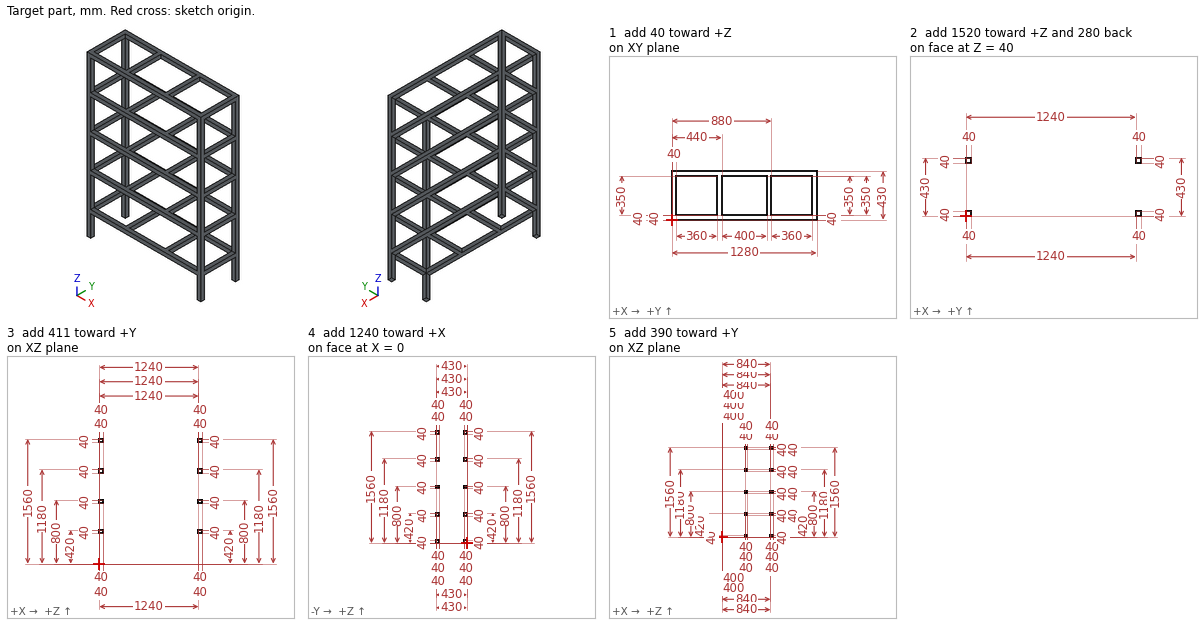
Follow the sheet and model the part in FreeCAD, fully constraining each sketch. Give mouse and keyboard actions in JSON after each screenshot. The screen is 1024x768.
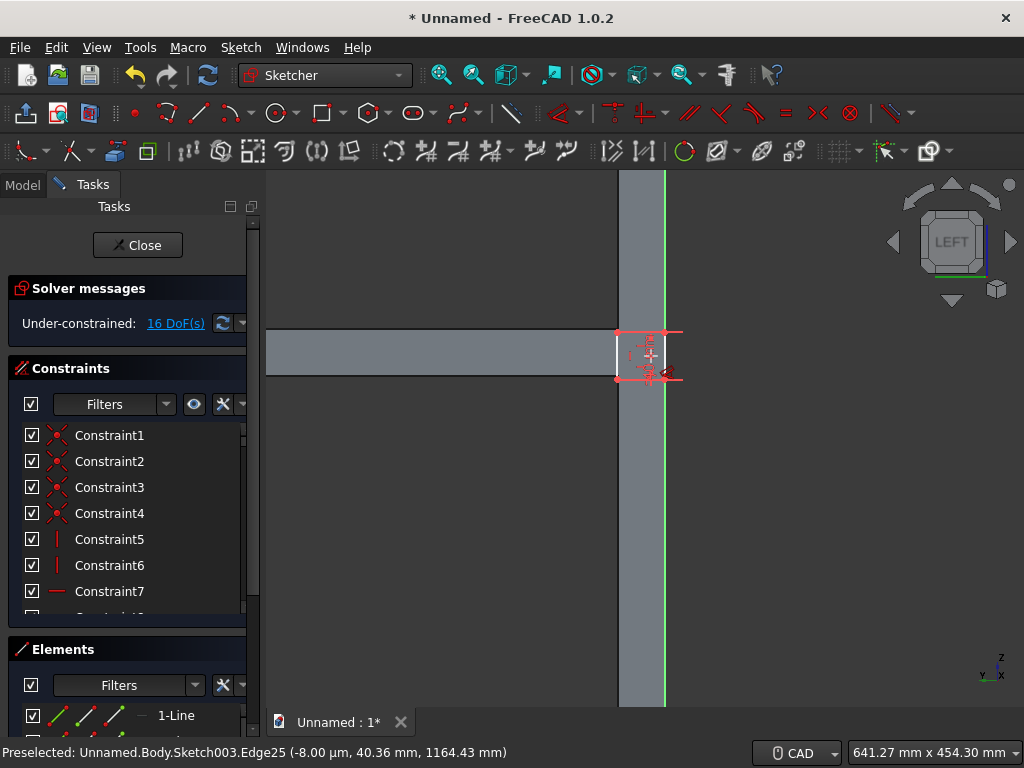
{"action": "left_click", "coordinate": [632, 380]}
{"action": "left_click", "coordinate": [641, 414]}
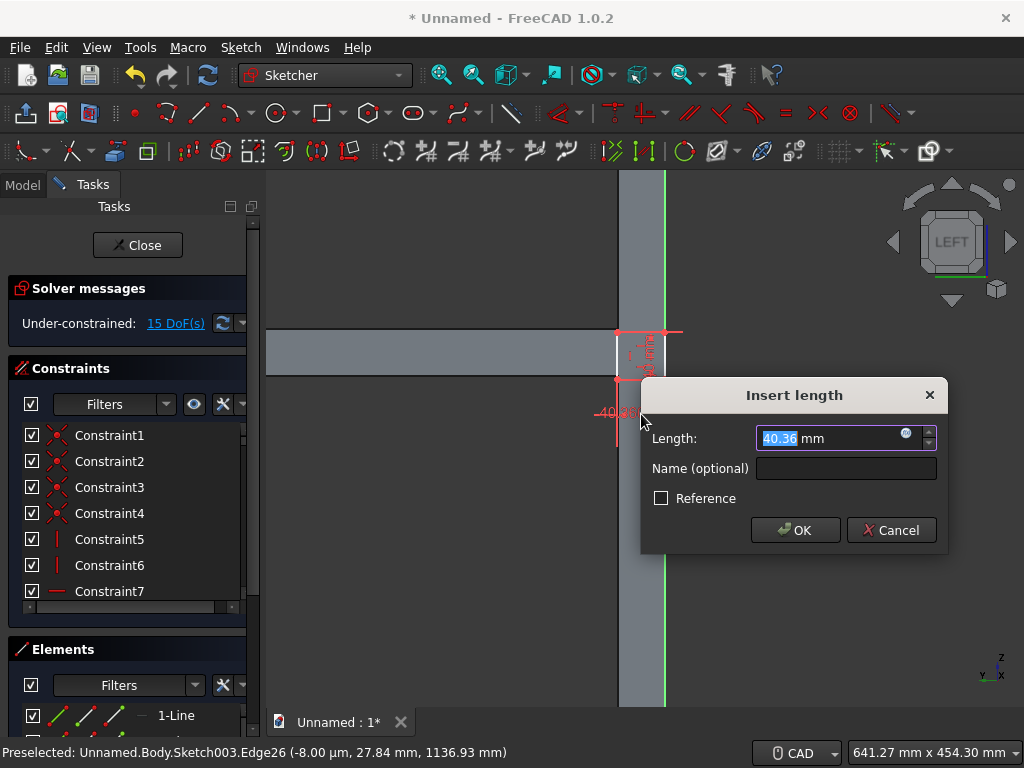
{"action": "type", "text": "40"}
{"action": "key", "text": "Return"}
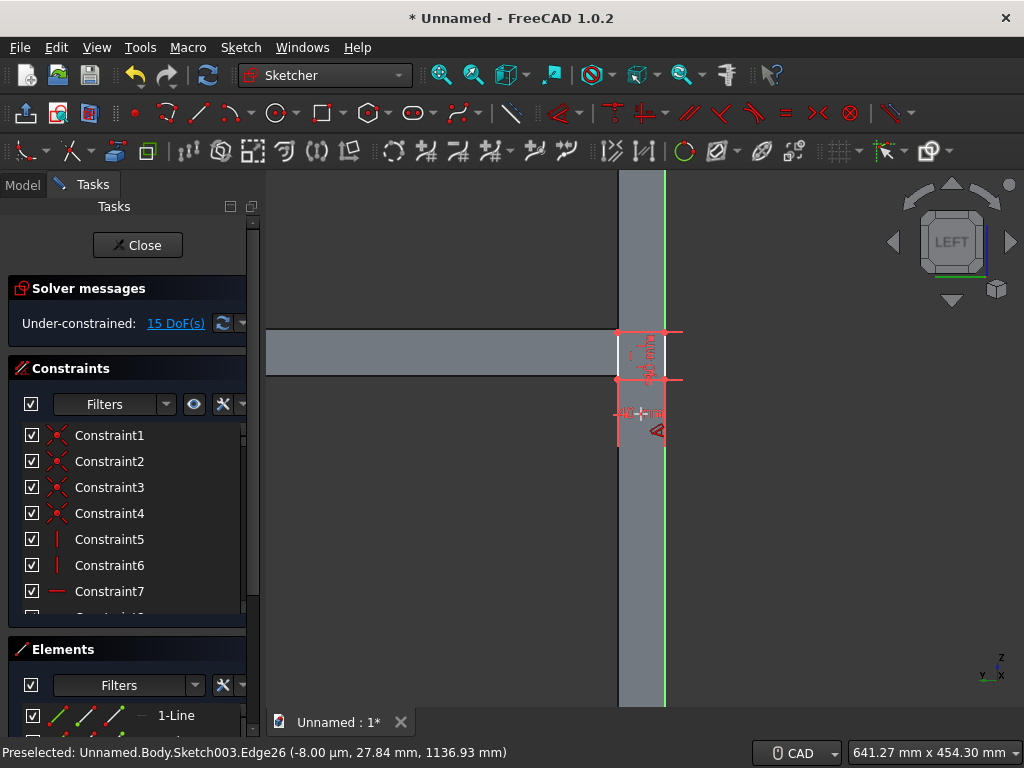
{"action": "scroll", "coordinate": [618, 347], "scroll_direction": "down", "scroll_amount": 8}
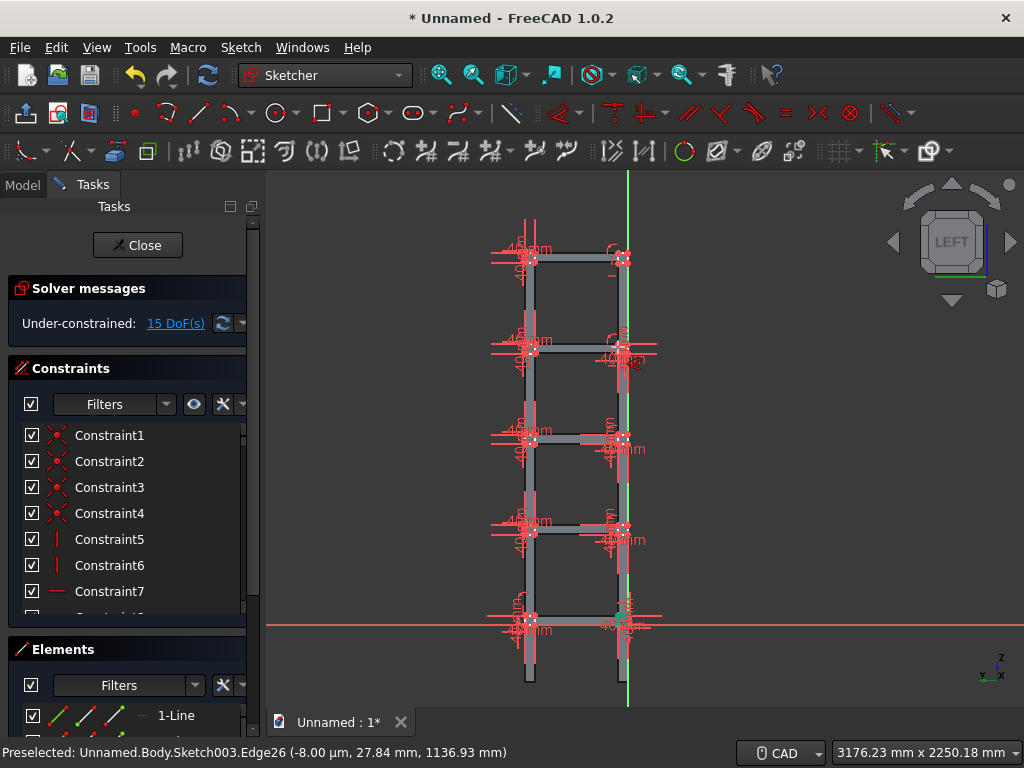
{"action": "scroll", "coordinate": [618, 256], "scroll_direction": "up", "scroll_amount": 8}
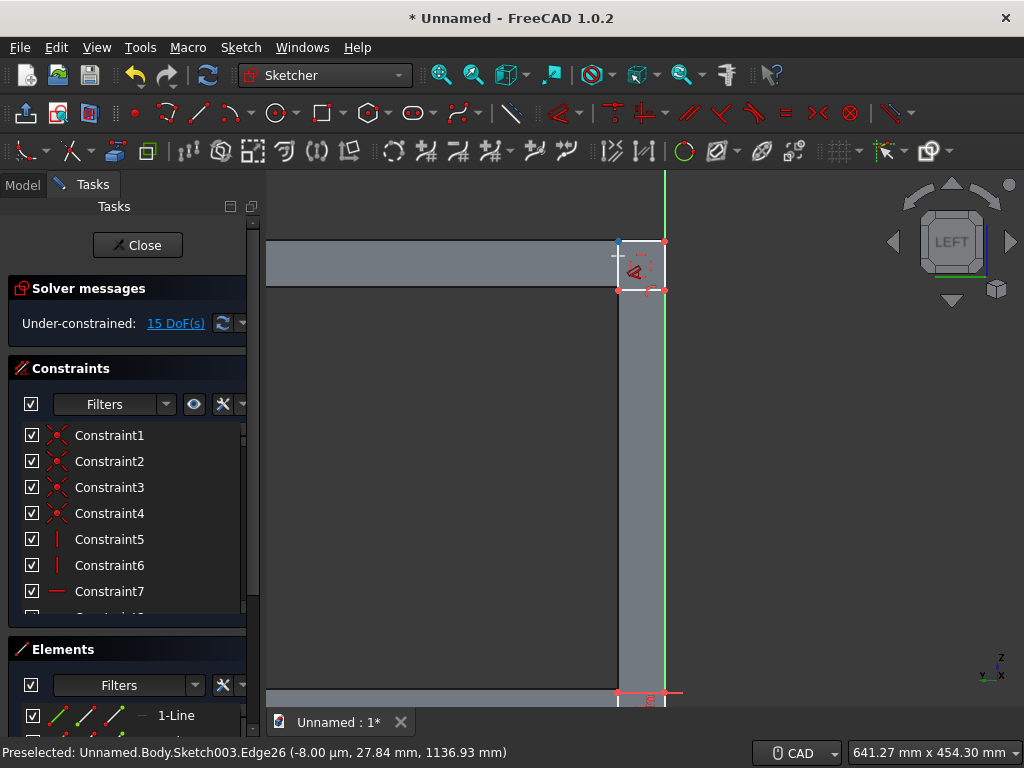
{"action": "left_click", "coordinate": [618, 256]}
{"action": "left_click", "coordinate": [584, 266]}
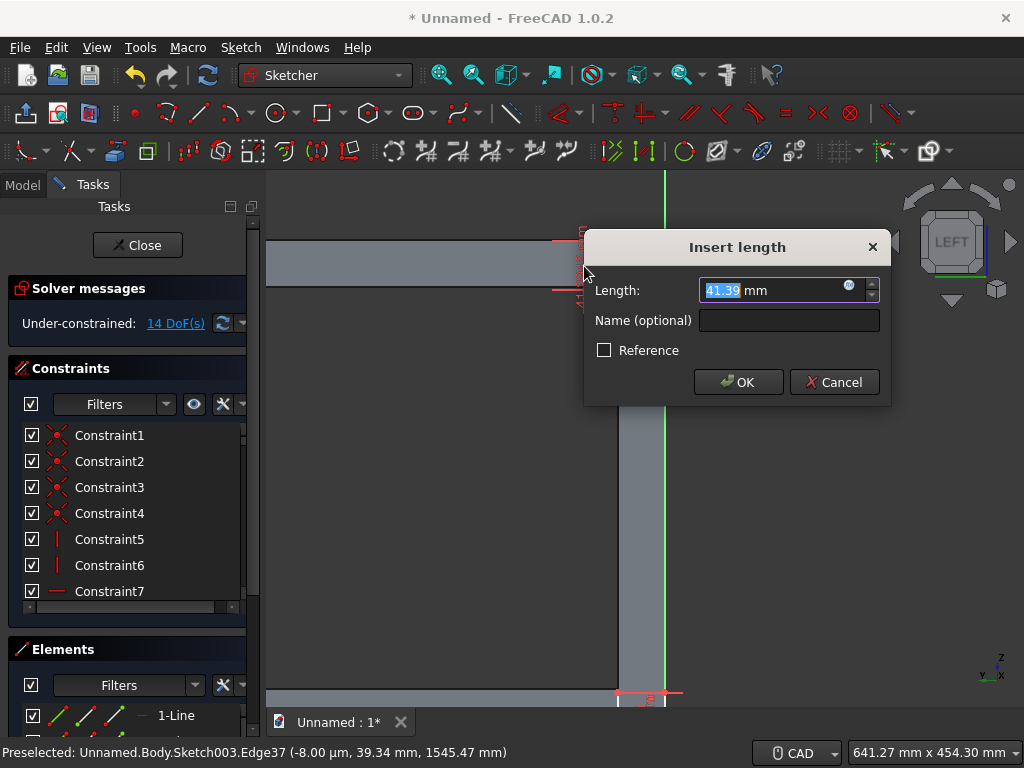
{"action": "type", "text": "40"}
{"action": "key", "text": "Return"}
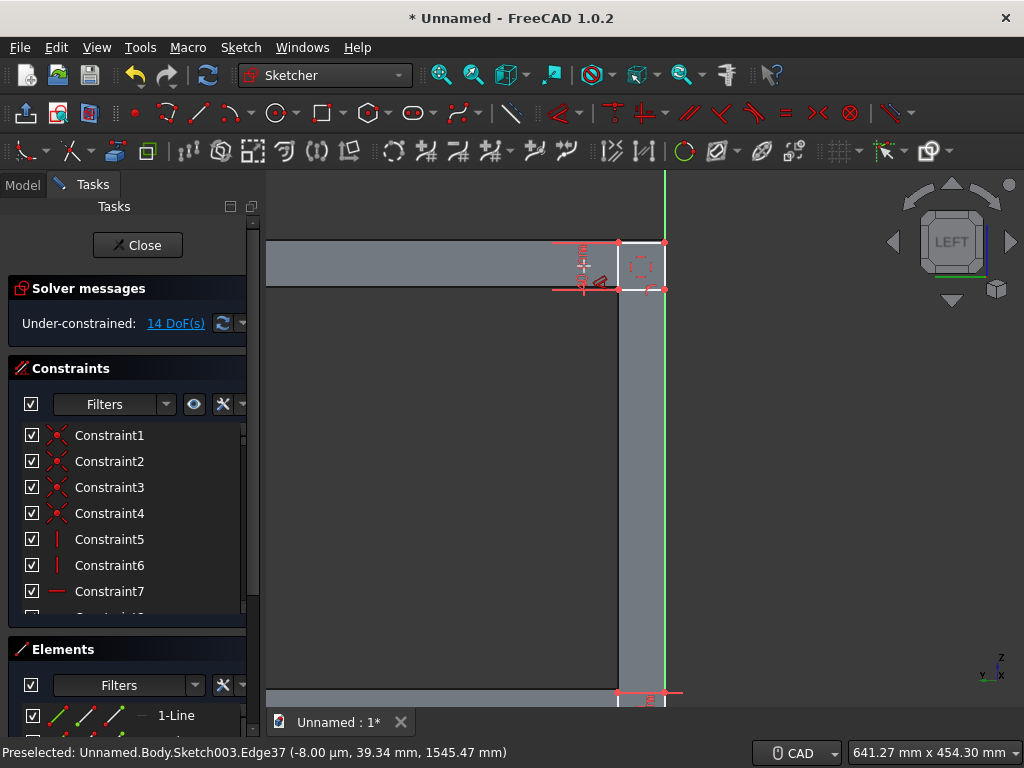
{"action": "left_click", "coordinate": [632, 290]}
{"action": "left_click", "coordinate": [642, 324]}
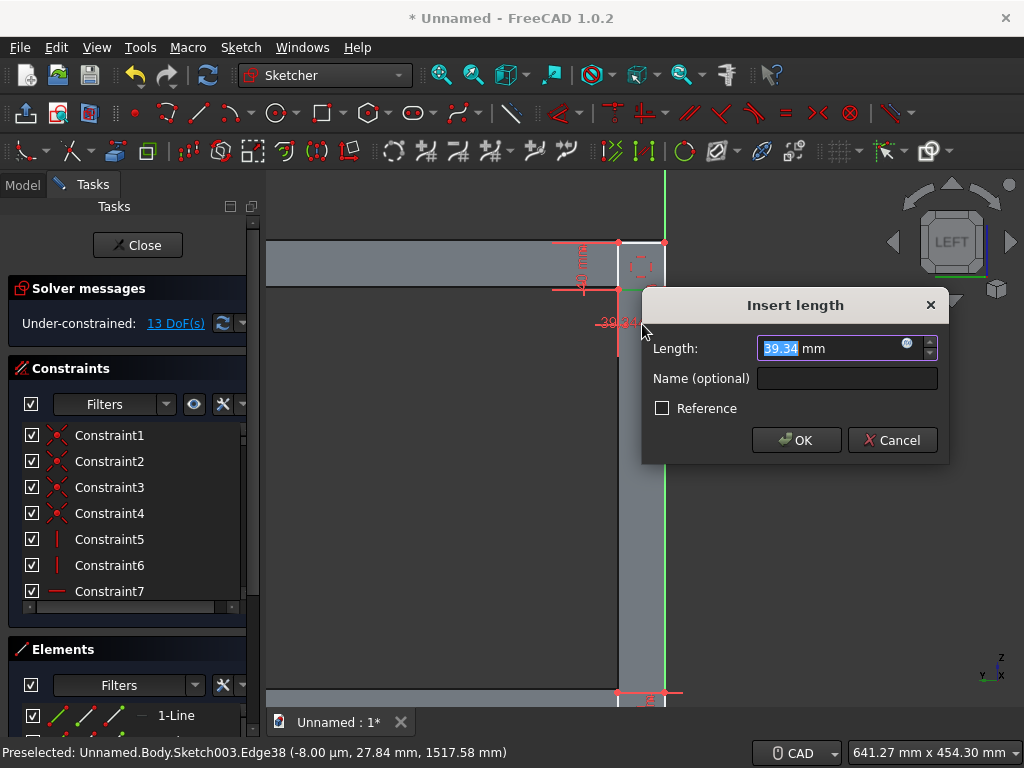
{"action": "type", "text": "40"}
{"action": "key", "text": "Return"}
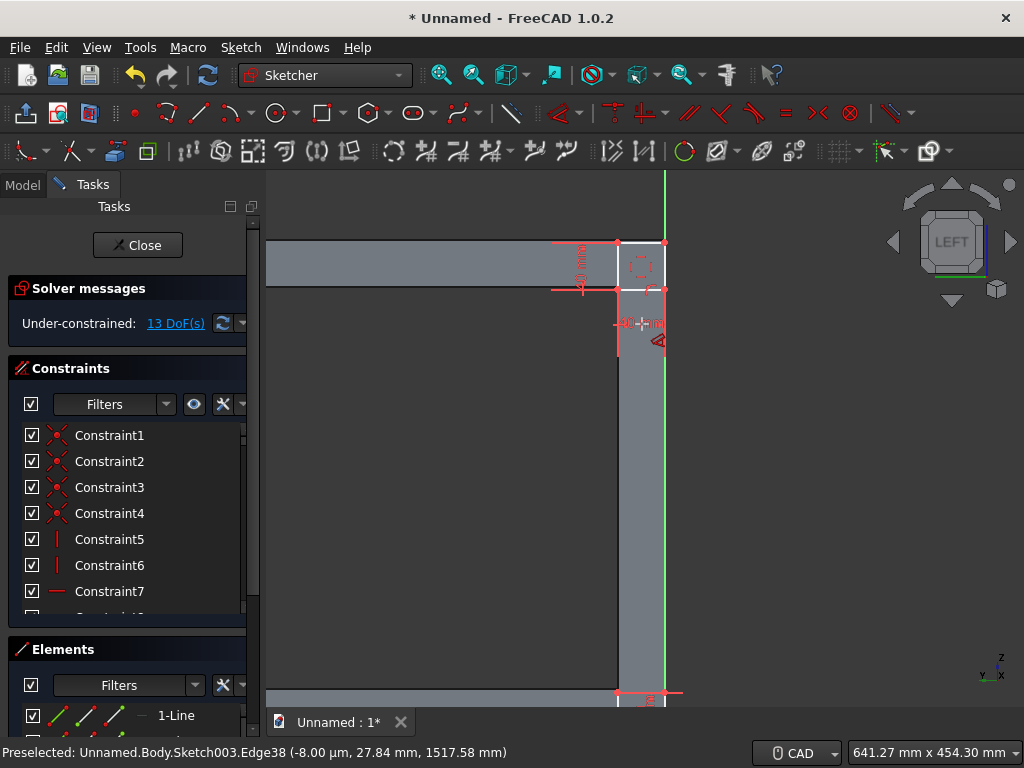
{"action": "scroll", "coordinate": [618, 256], "scroll_direction": "down", "scroll_amount": 8}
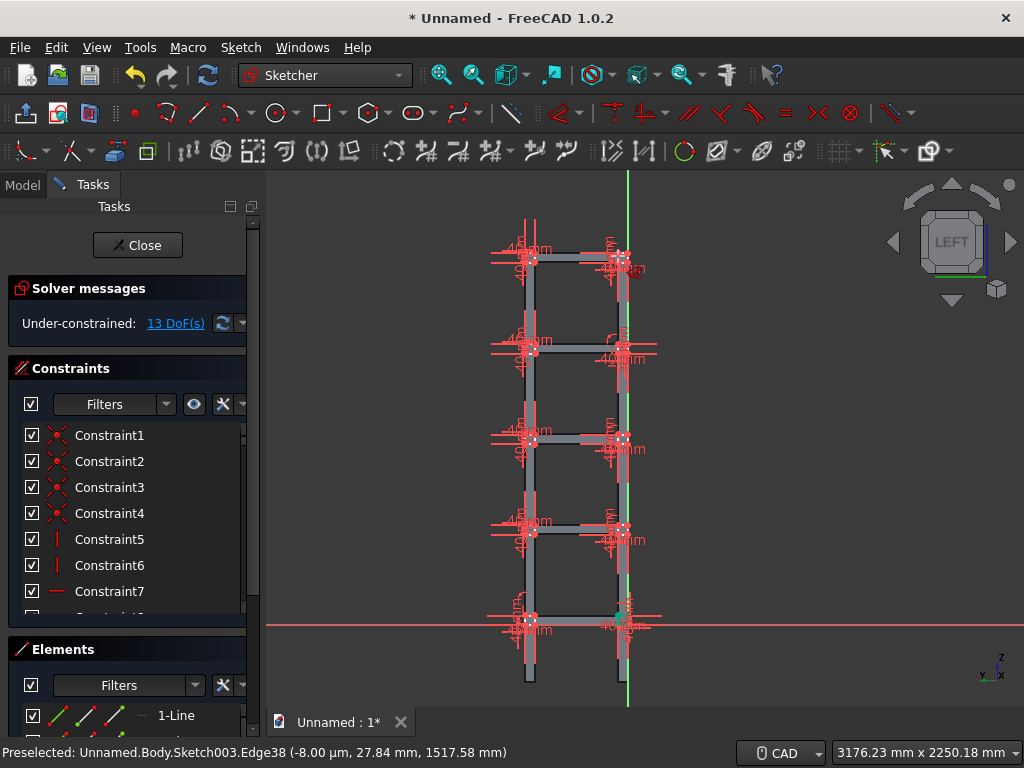
{"action": "scroll", "coordinate": [525, 616], "scroll_direction": "up", "scroll_amount": 2}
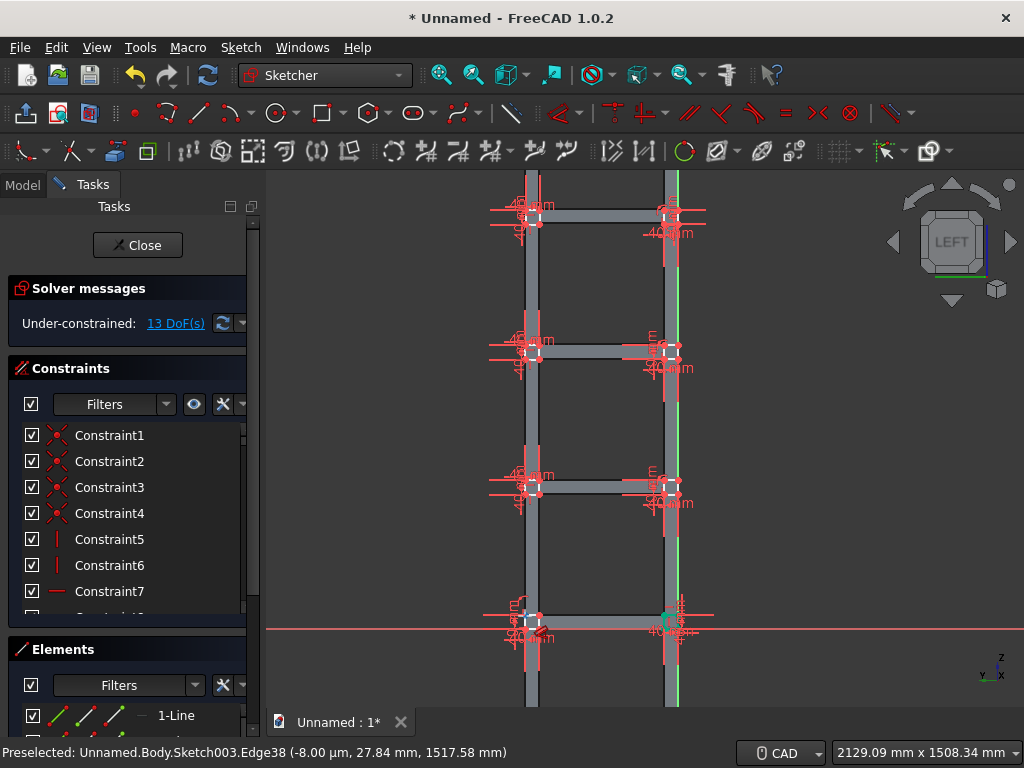
{"action": "left_click", "coordinate": [525, 615]}
{"action": "left_click", "coordinate": [602, 663]}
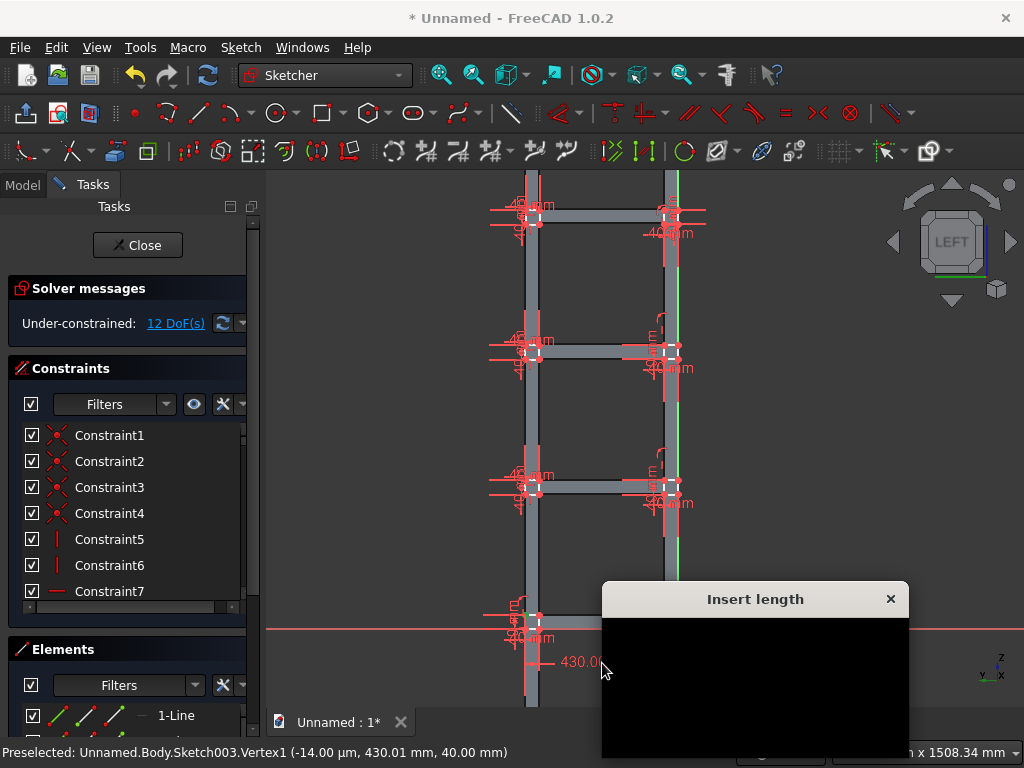
{"action": "type", "text": "430"}
{"action": "key", "text": "Return"}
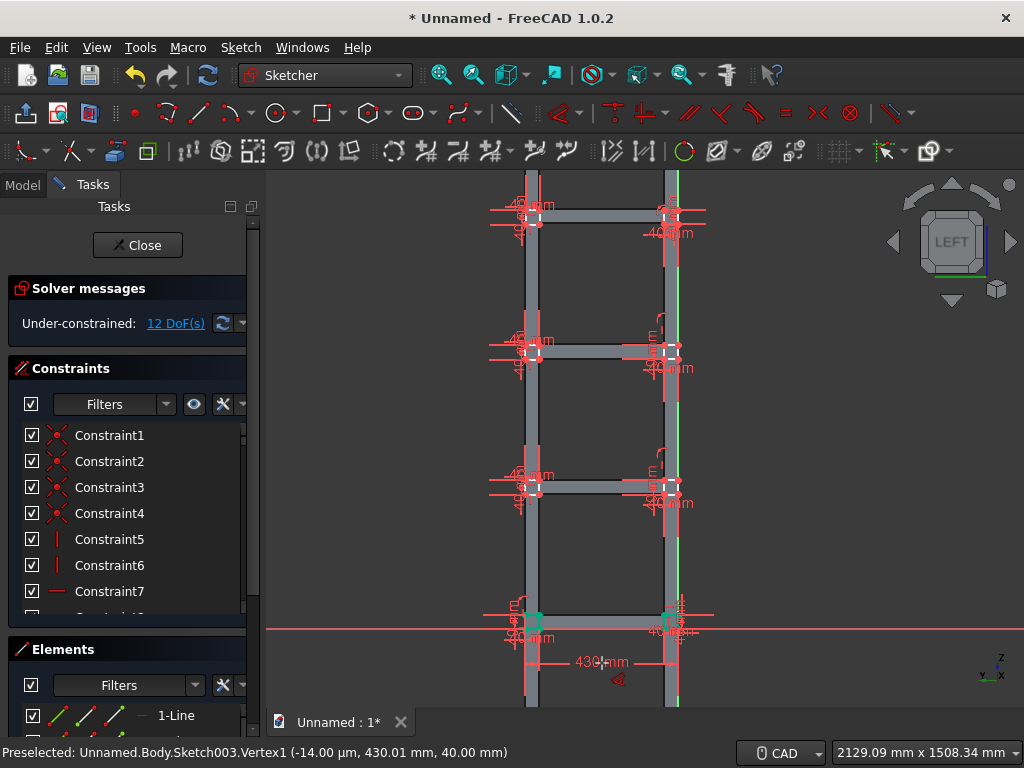
{"action": "left_click", "coordinate": [664, 480]}
{"action": "left_click", "coordinate": [712, 555]}